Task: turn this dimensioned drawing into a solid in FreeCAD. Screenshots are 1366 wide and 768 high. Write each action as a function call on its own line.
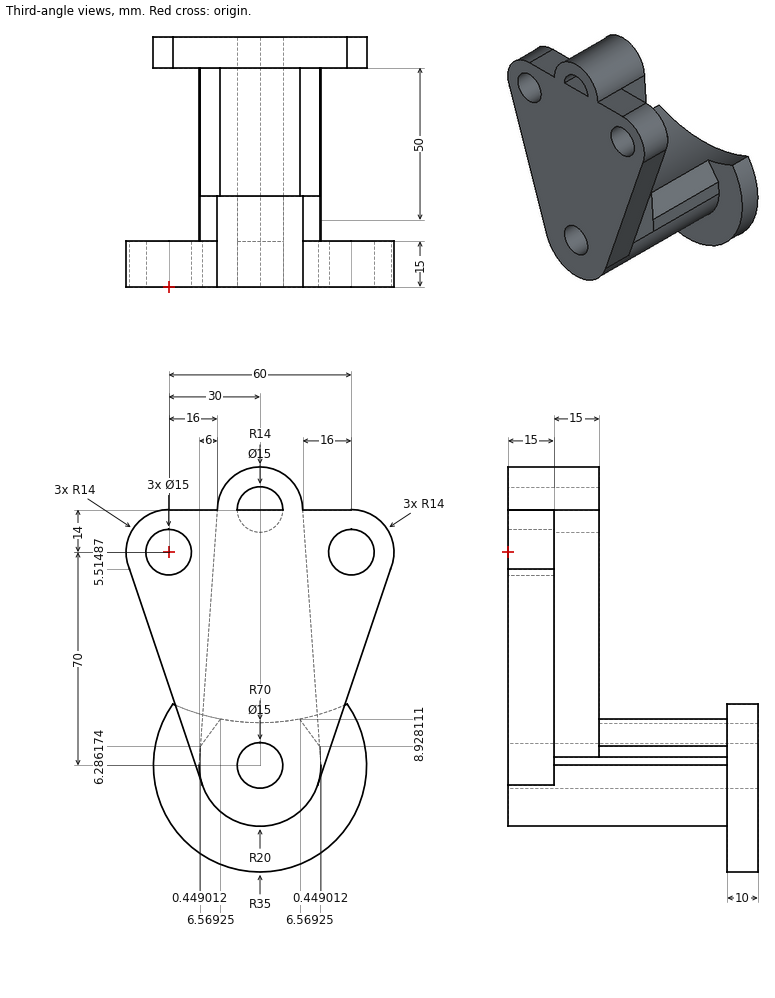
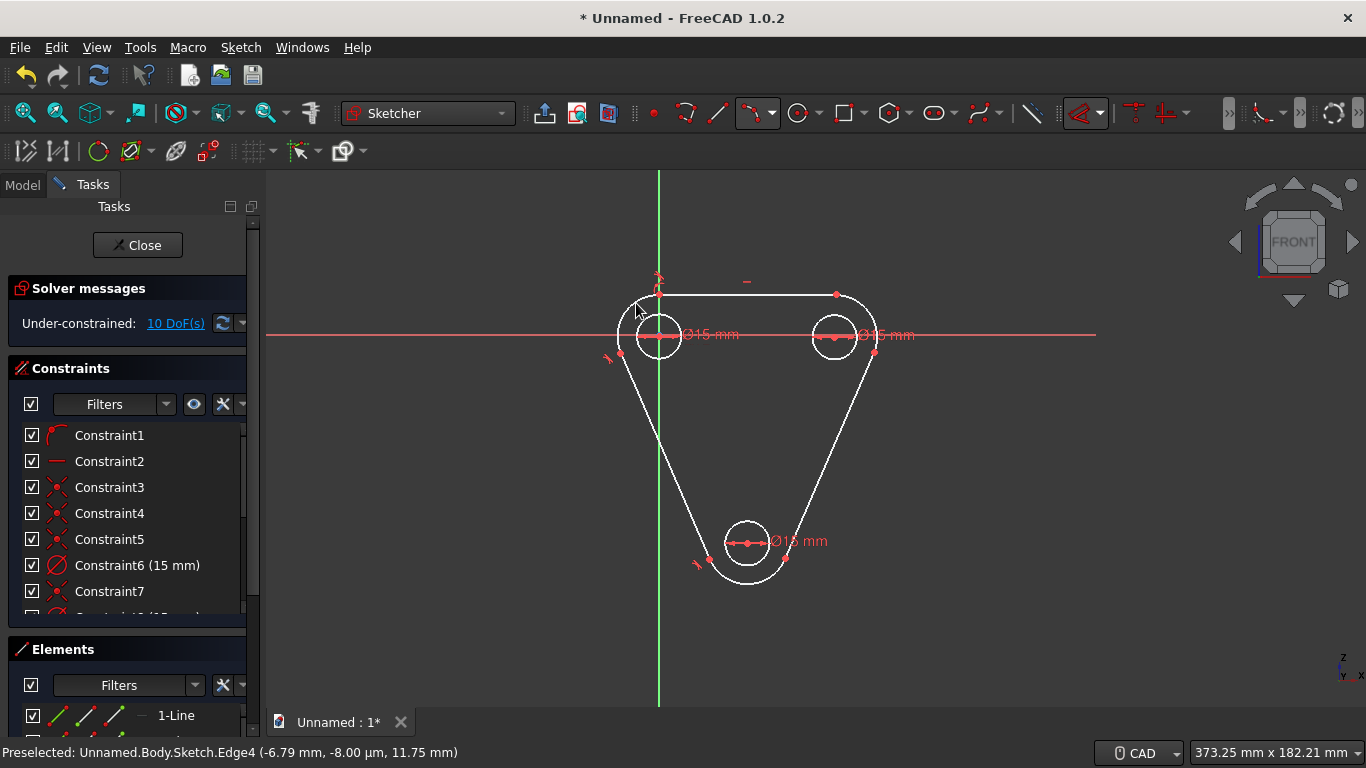
click(712, 295)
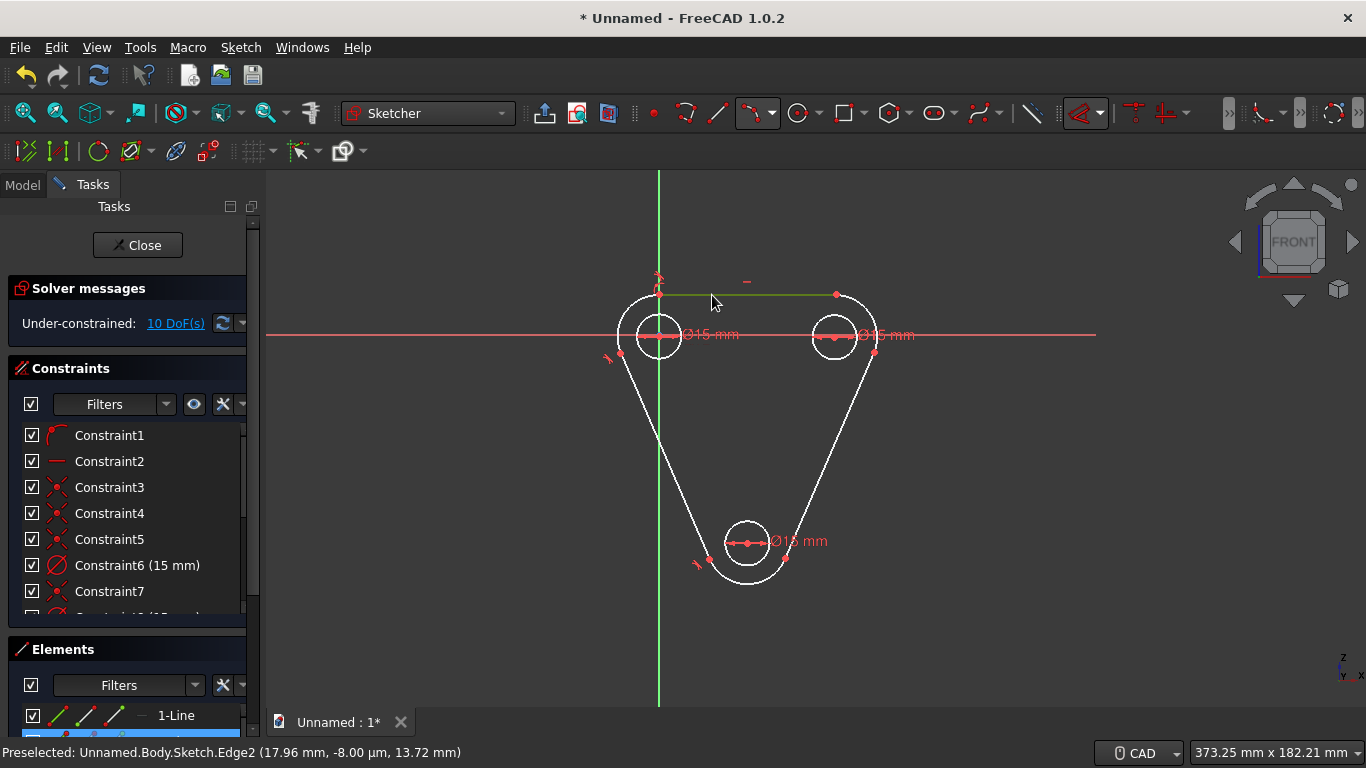
click(859, 303)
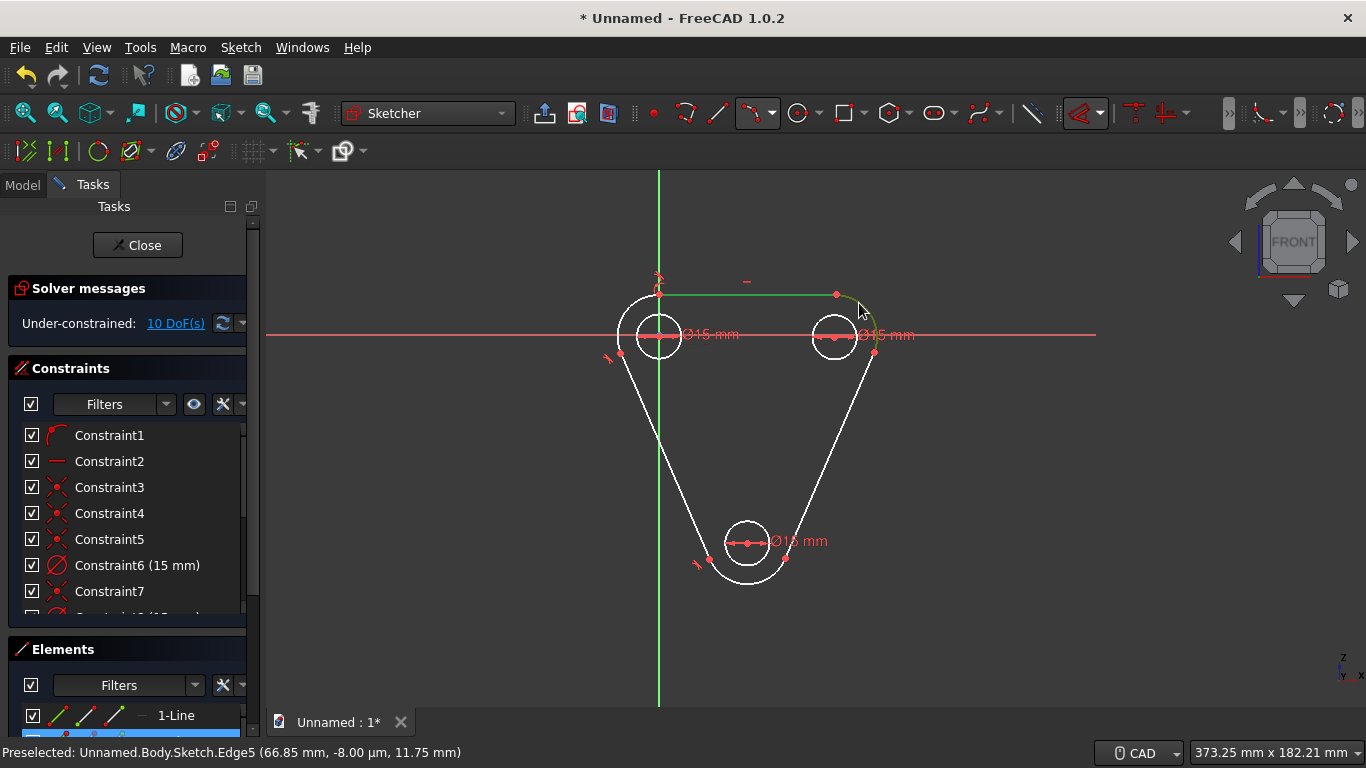
key(t)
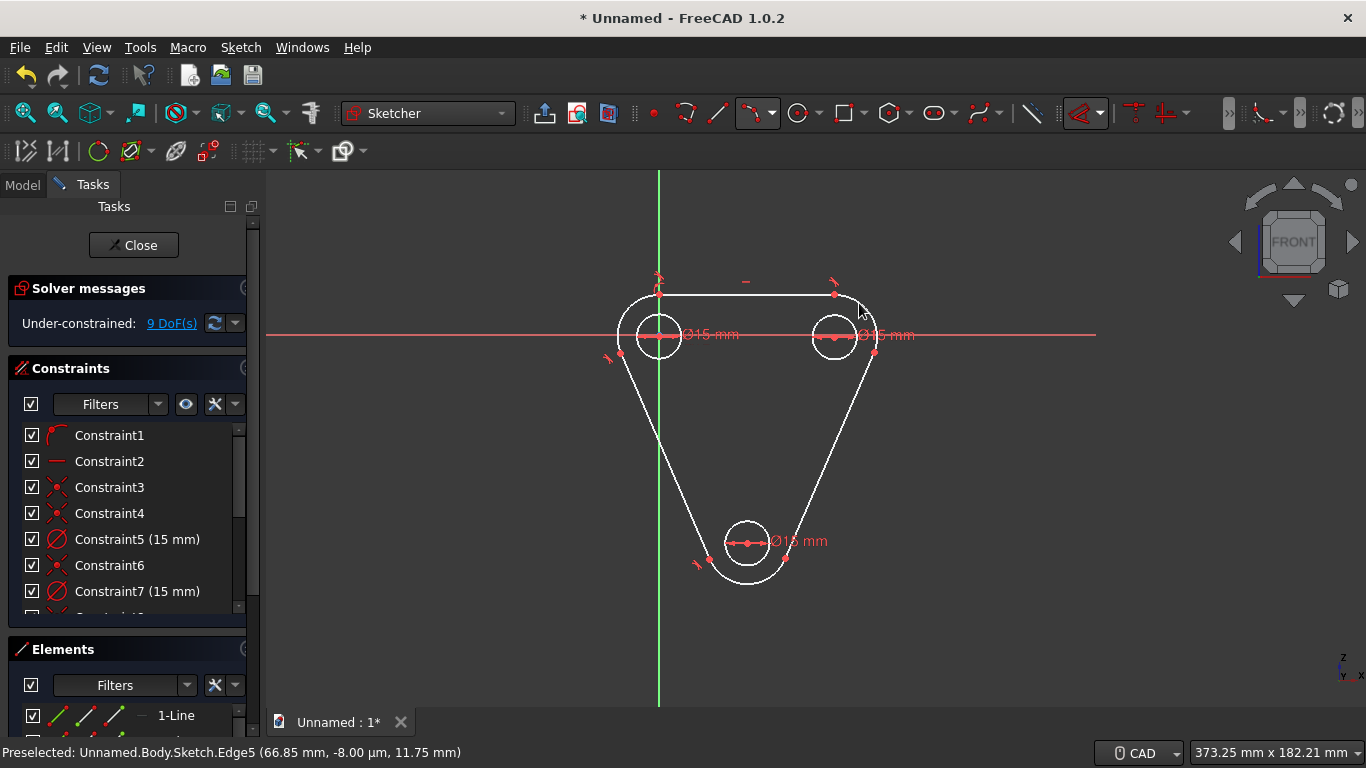
click(847, 415)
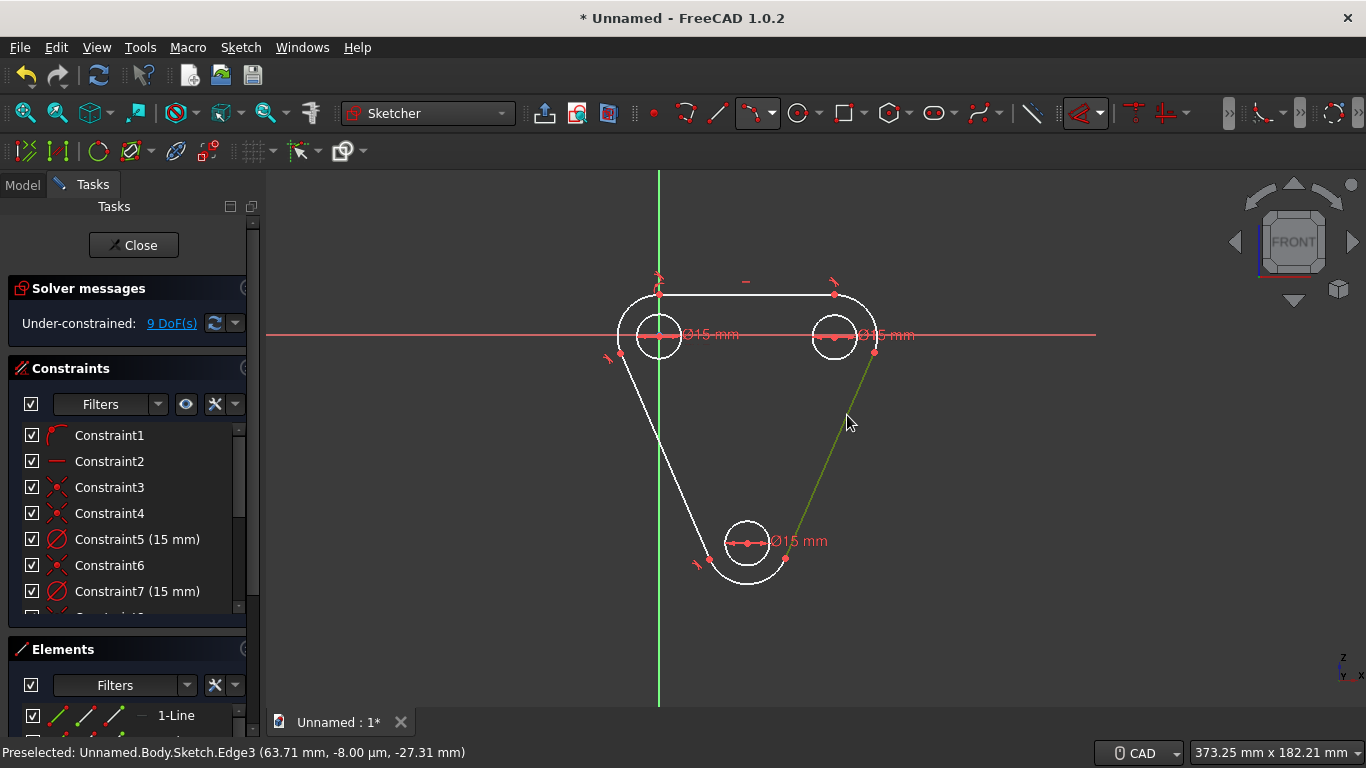
click(858, 302)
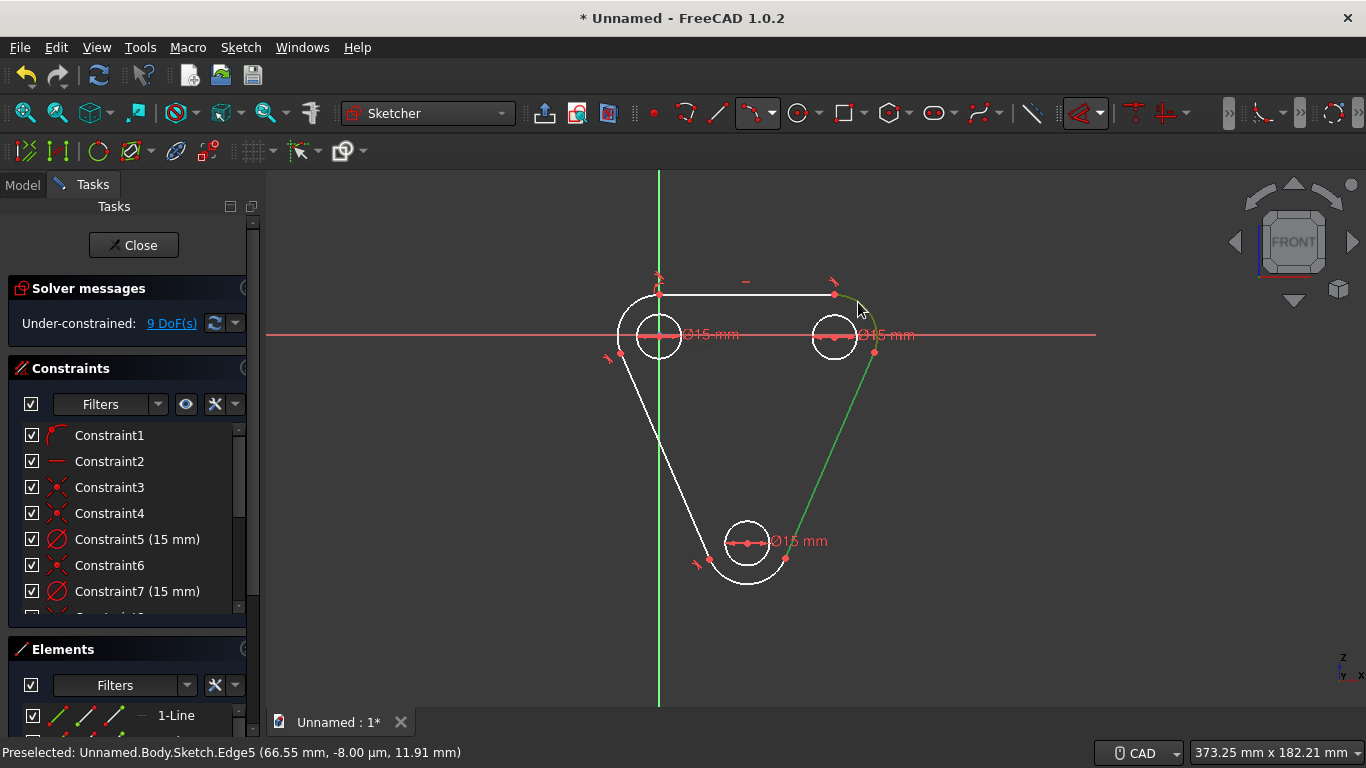
key(t)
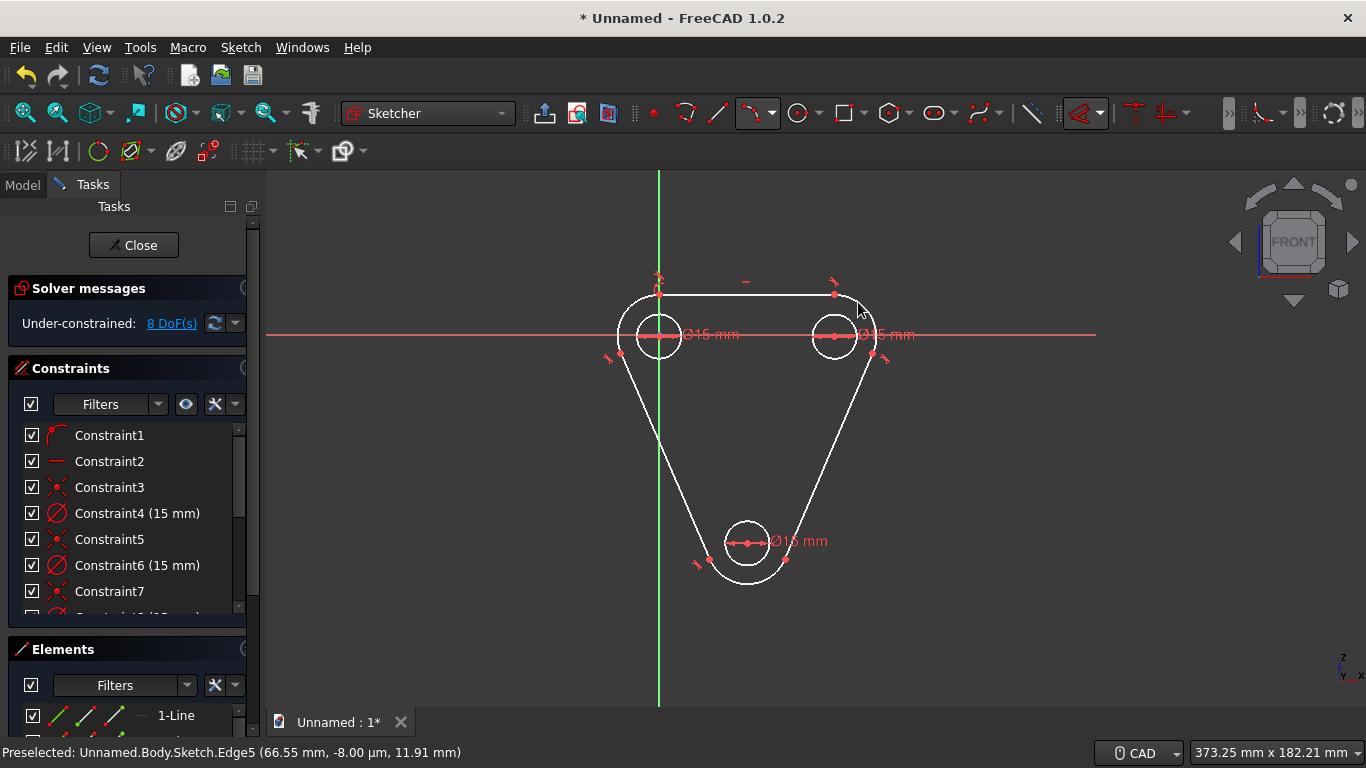
click(847, 415)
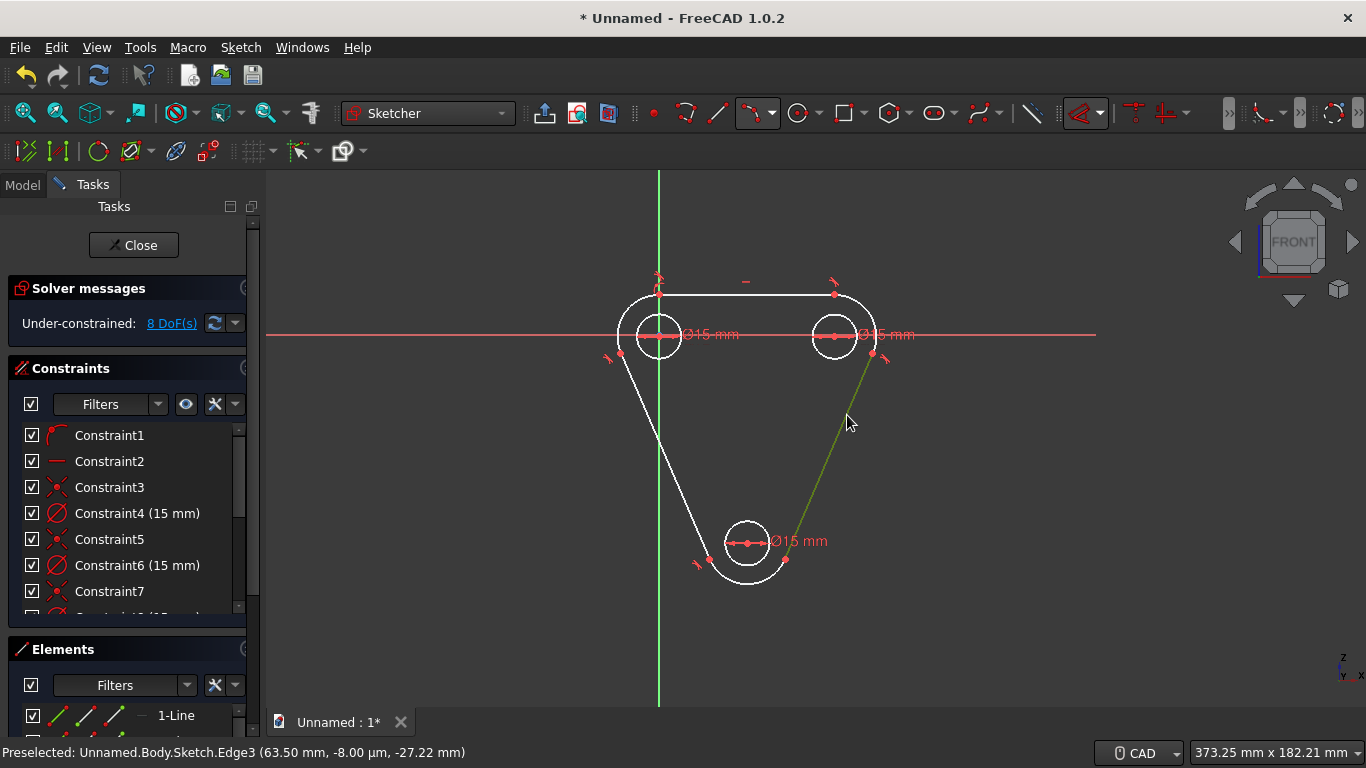
click(729, 580)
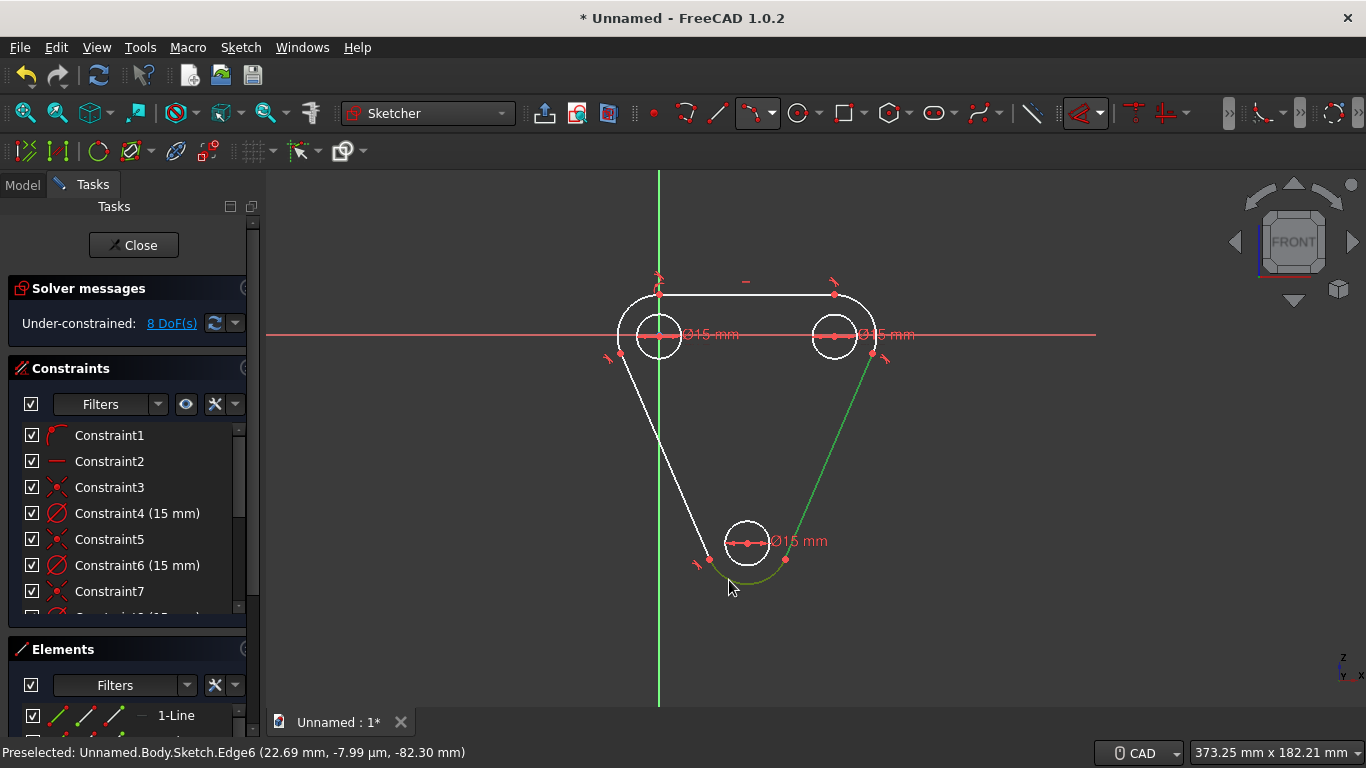
key(t)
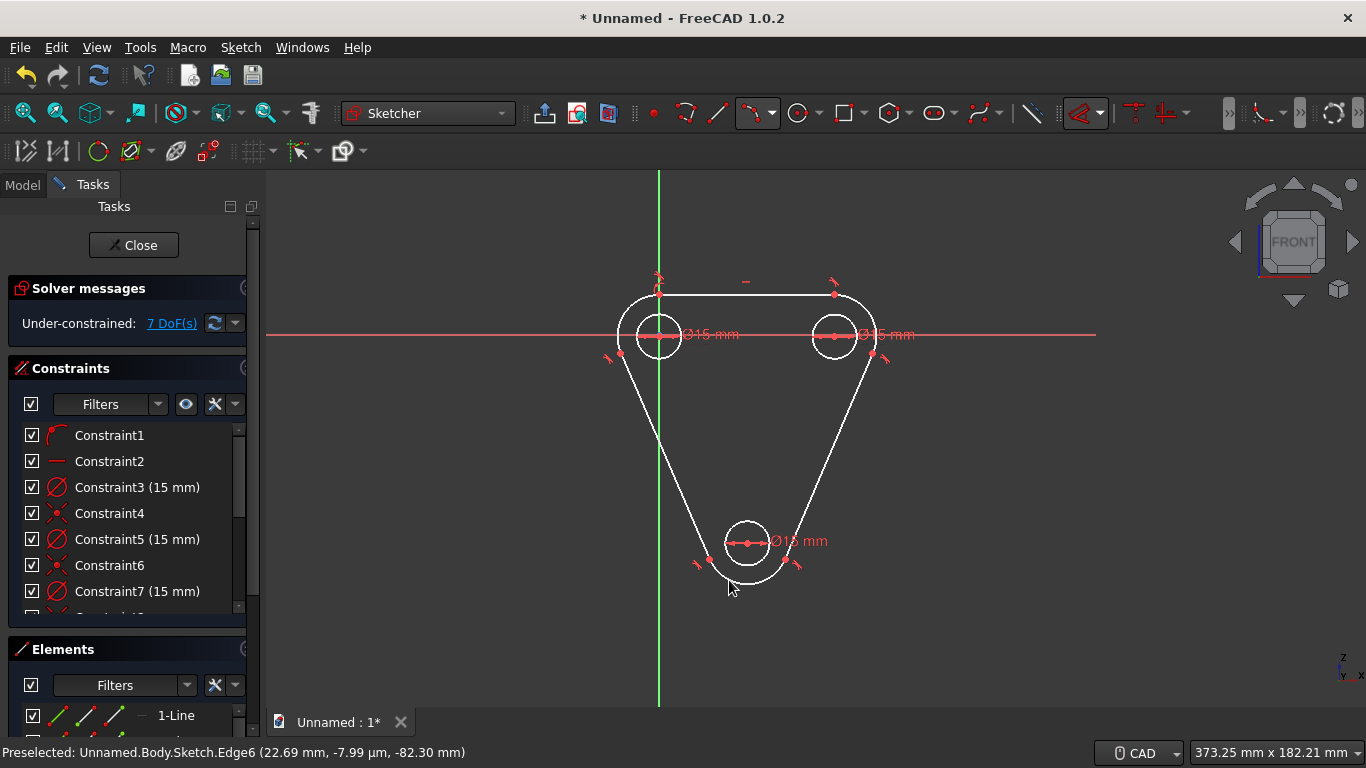
click(636, 302)